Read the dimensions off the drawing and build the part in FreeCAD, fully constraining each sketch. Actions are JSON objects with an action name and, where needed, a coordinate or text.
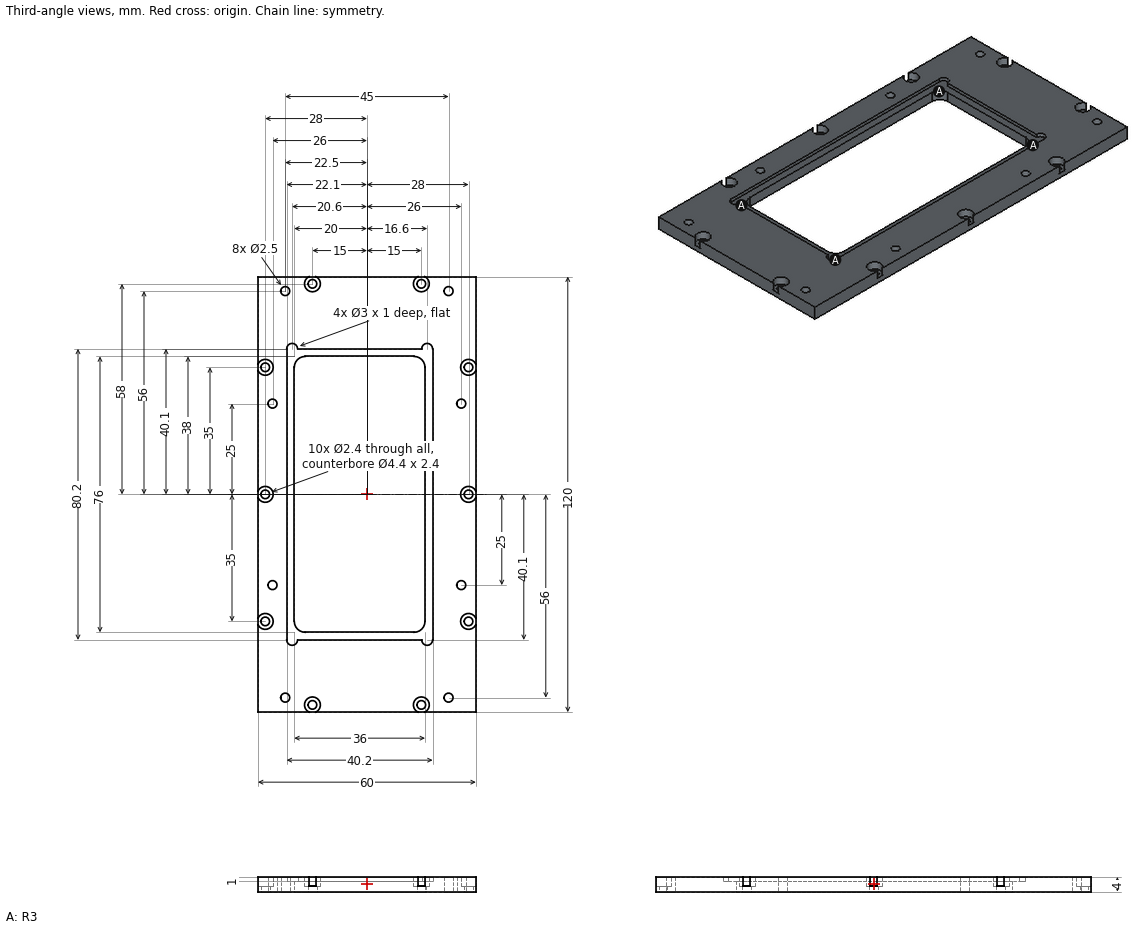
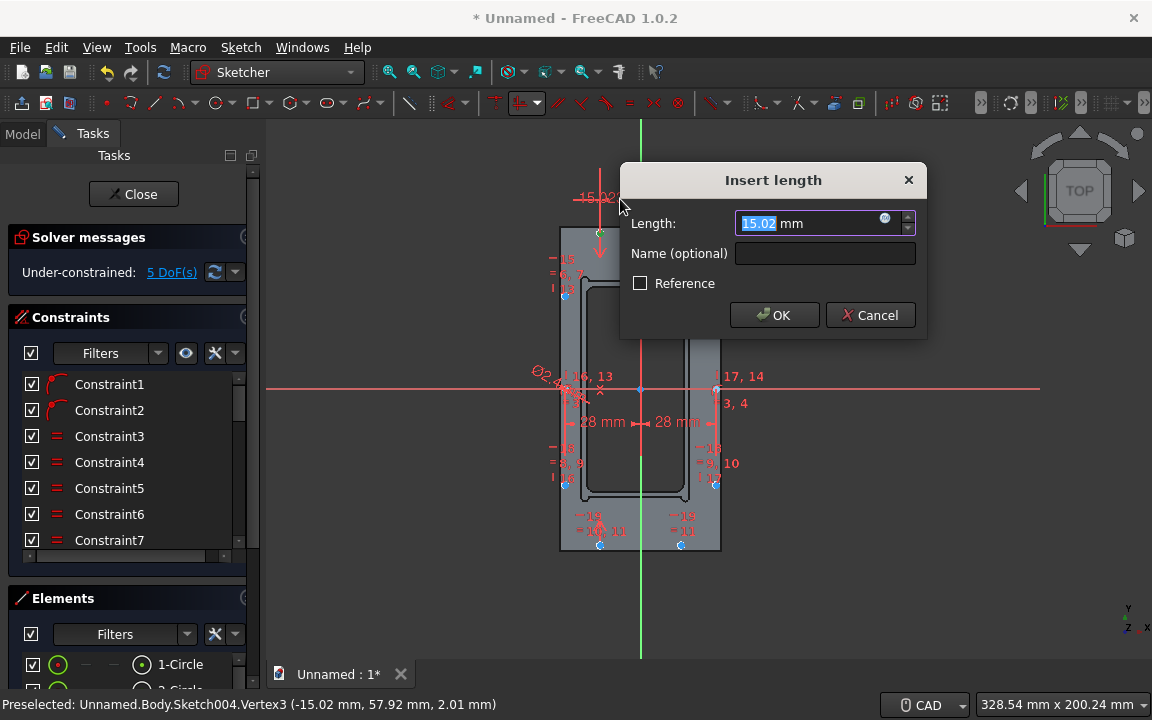
{"action": "type", "text": "15"}
{"action": "key", "text": "Return"}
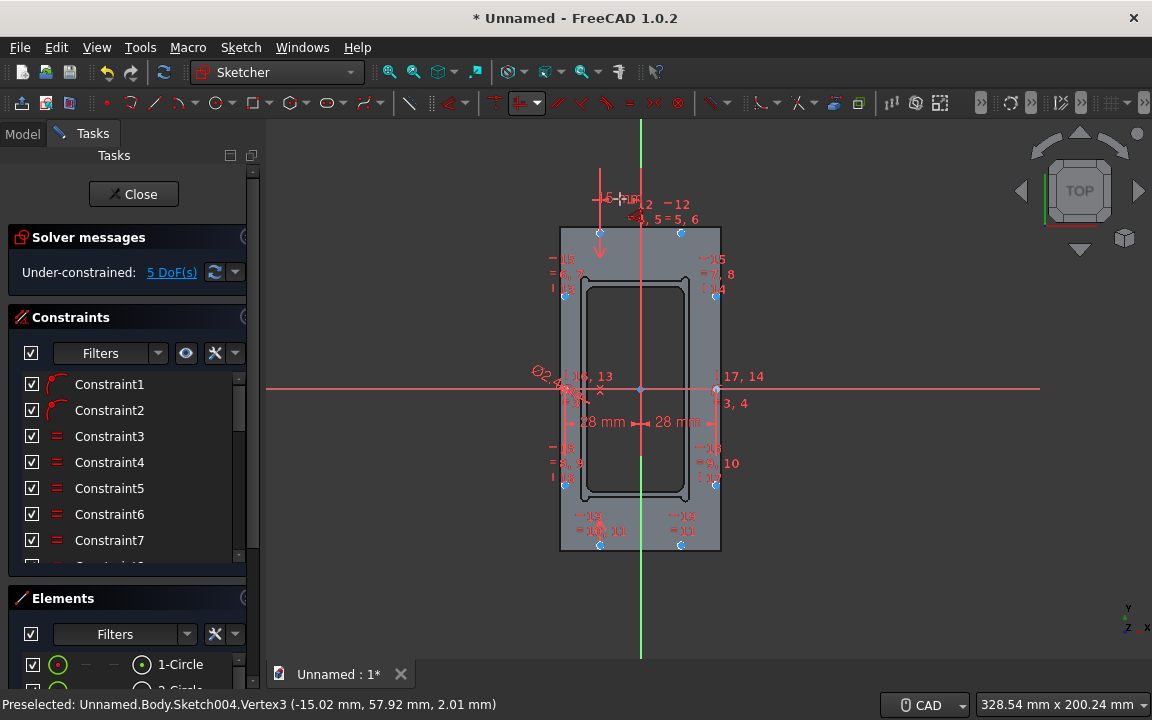
{"action": "left_click", "coordinate": [600, 233]}
{"action": "left_click", "coordinate": [566, 275]}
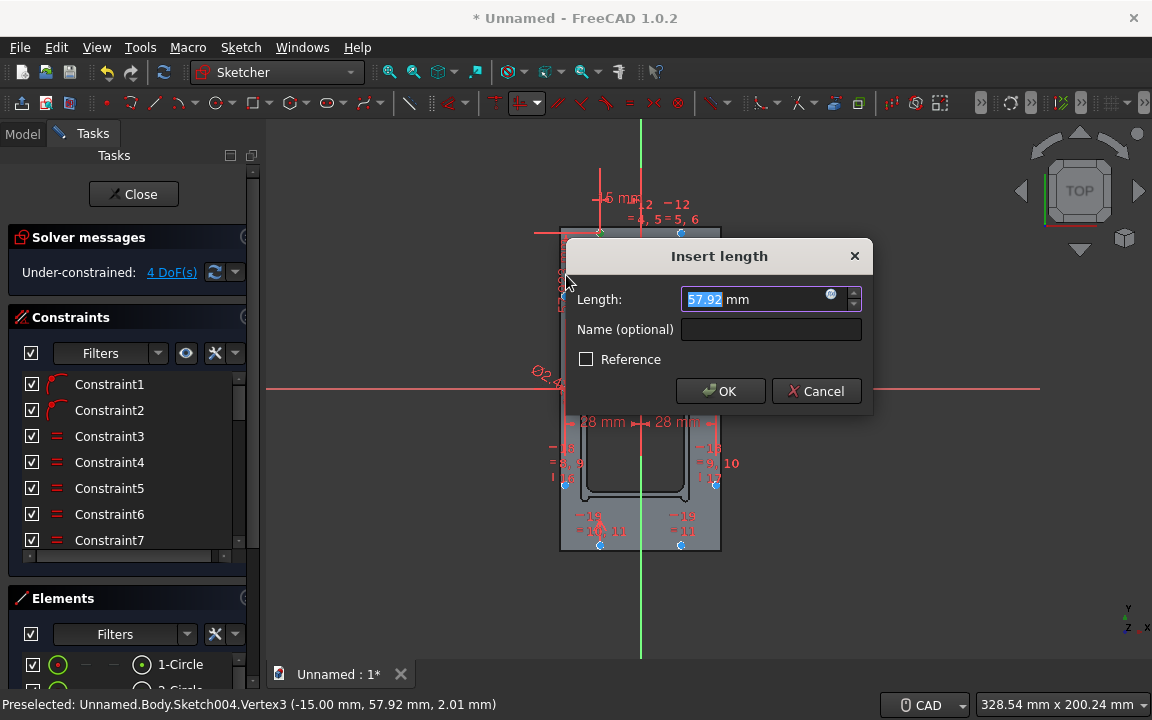
{"action": "type", "text": "58"}
{"action": "key", "text": "Return"}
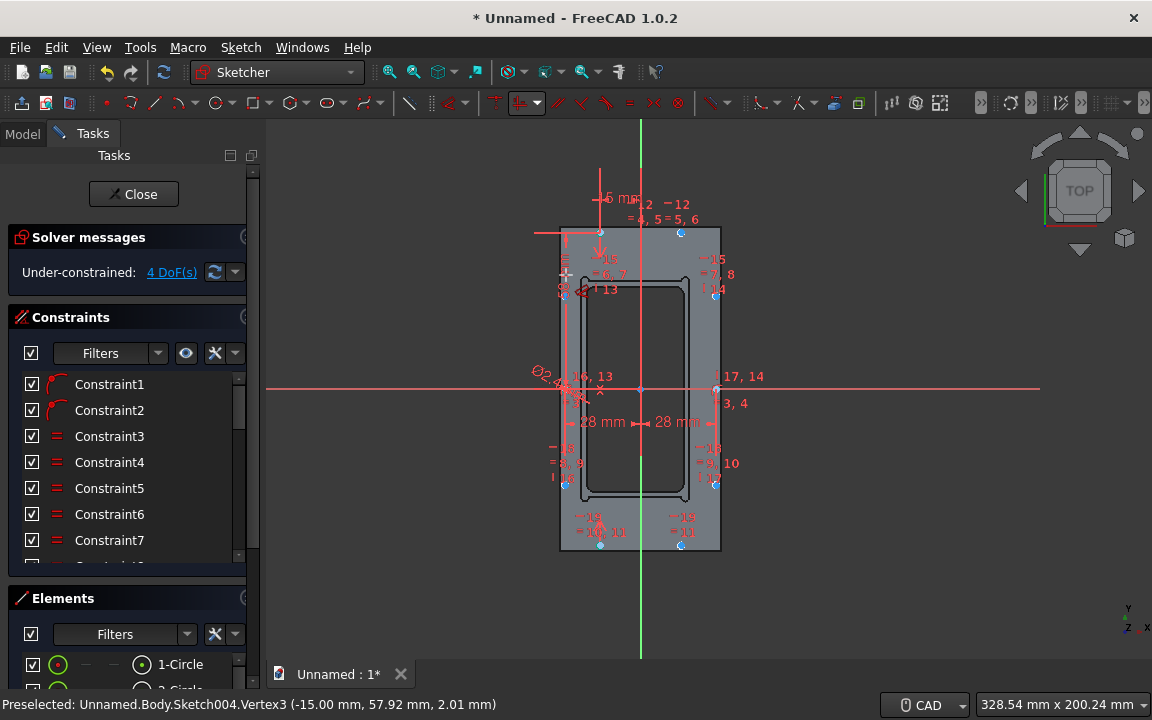
{"action": "left_click", "coordinate": [681, 233]}
{"action": "left_click", "coordinate": [661, 175]}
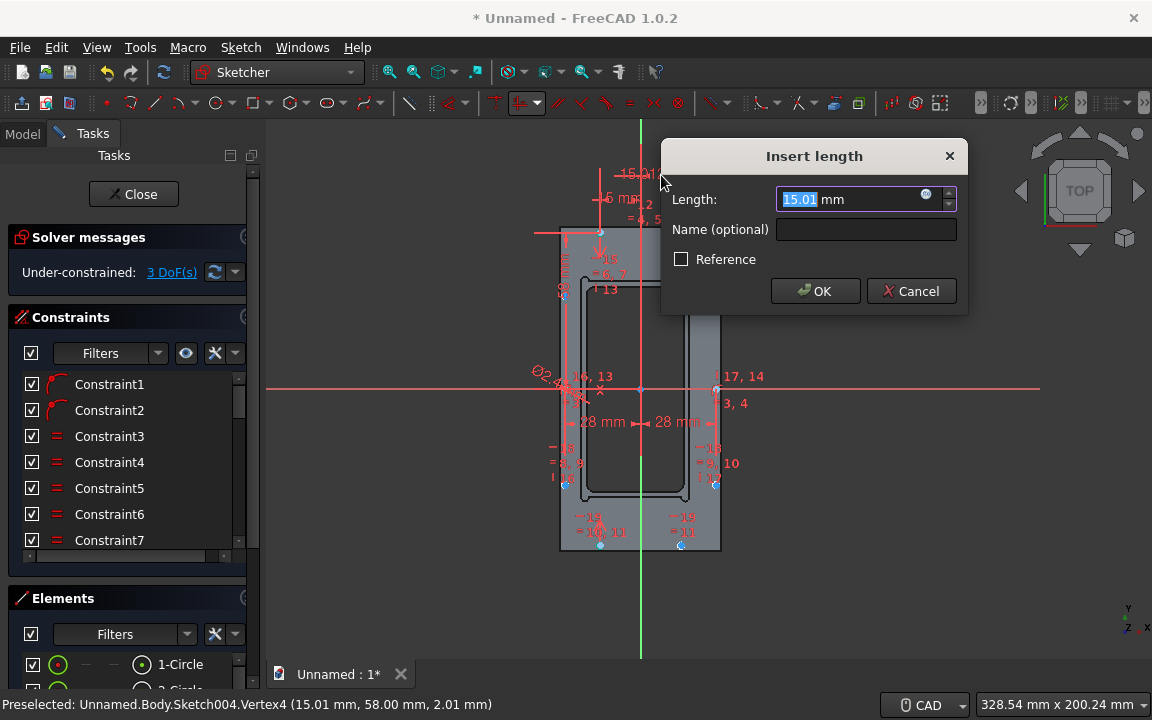
{"action": "type", "text": "15"}
{"action": "key", "text": "Return"}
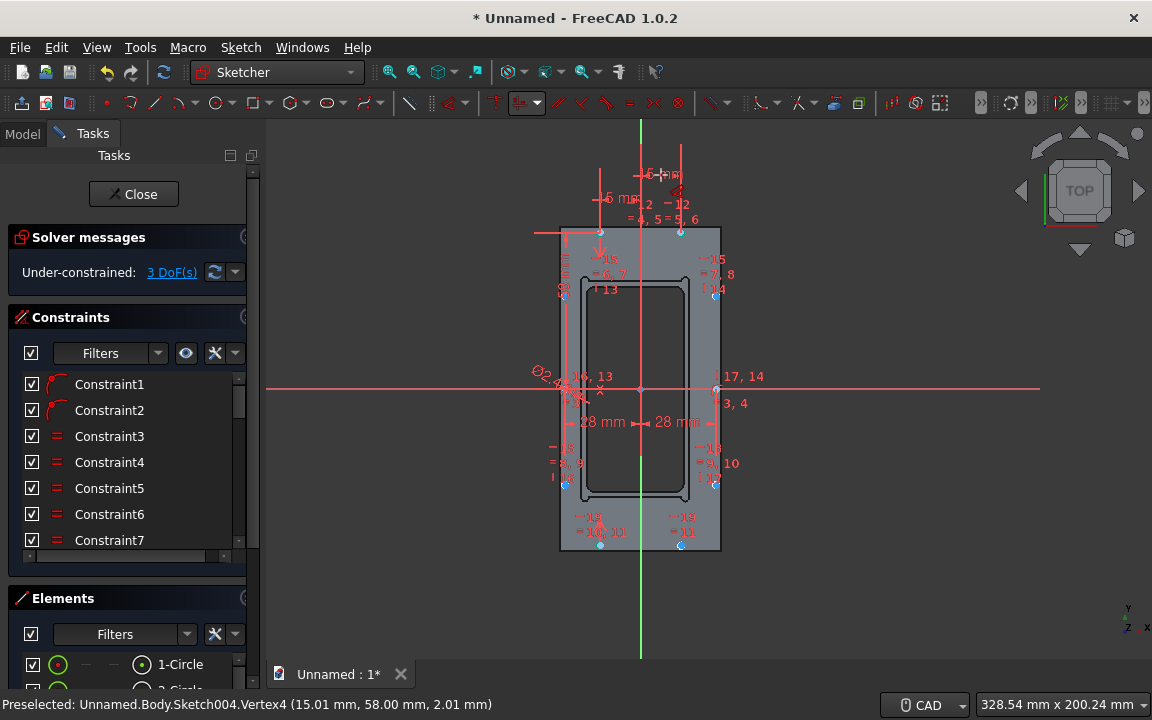
{"action": "left_click", "coordinate": [565, 296]}
{"action": "left_click", "coordinate": [531, 343]}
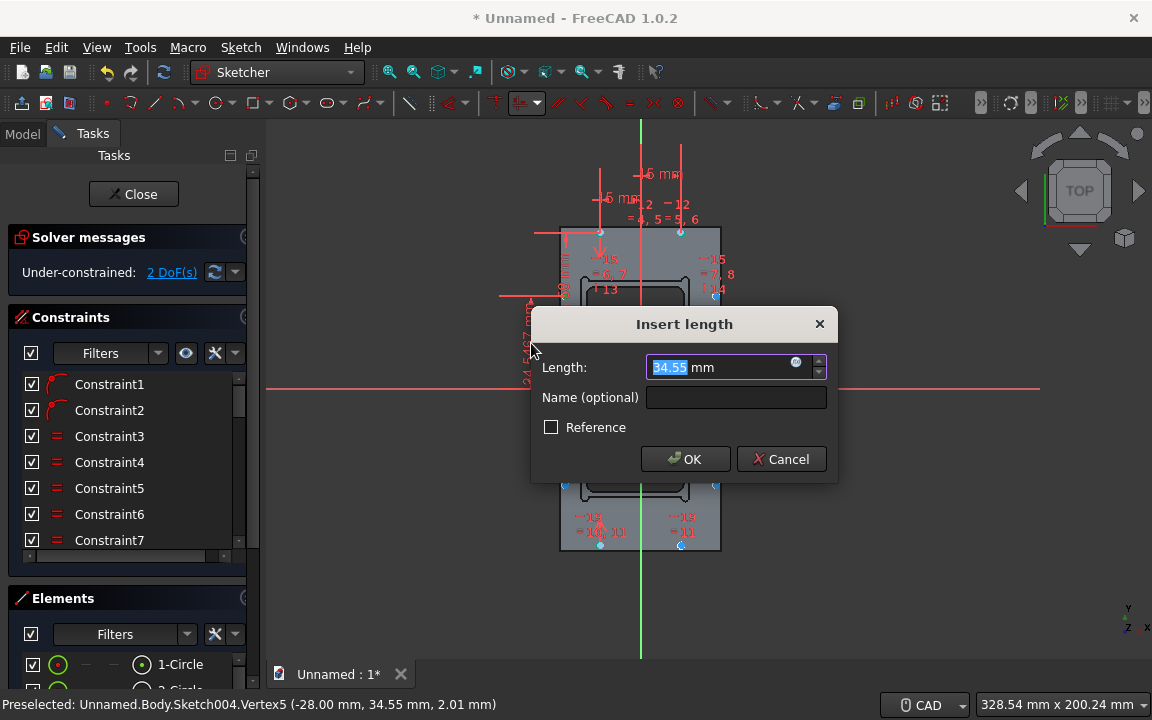
{"action": "type", "text": "35"}
{"action": "key", "text": "Return"}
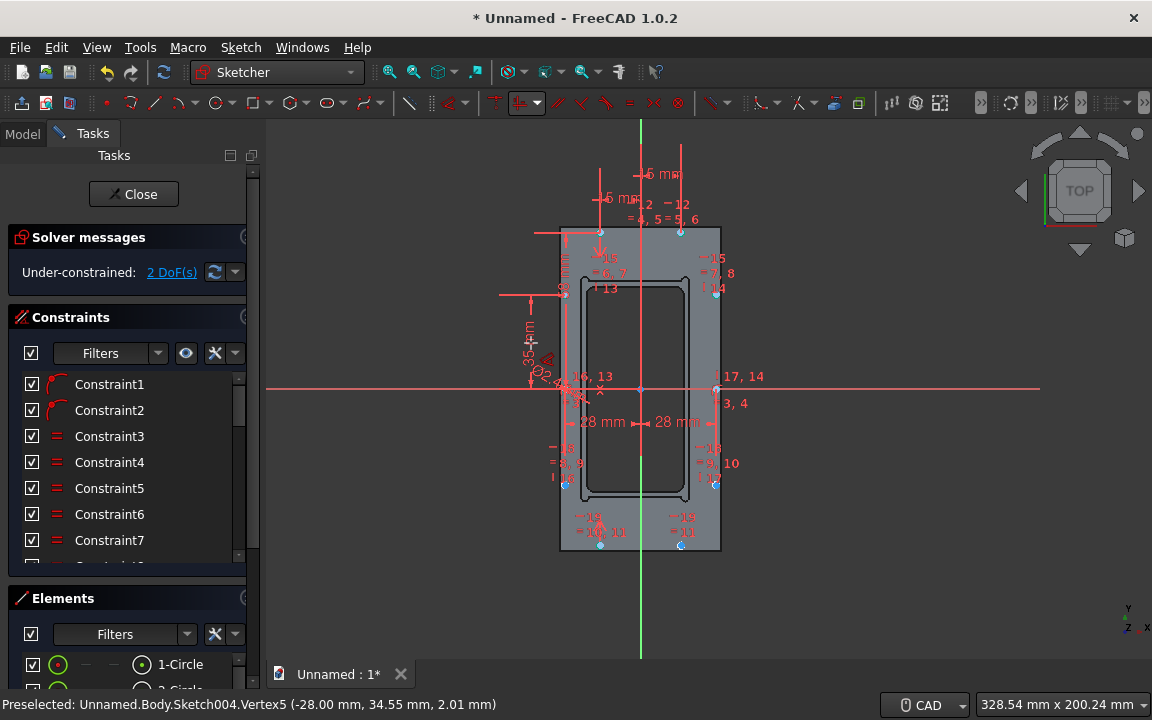
{"action": "left_click", "coordinate": [565, 485]}
{"action": "left_click", "coordinate": [531, 437]}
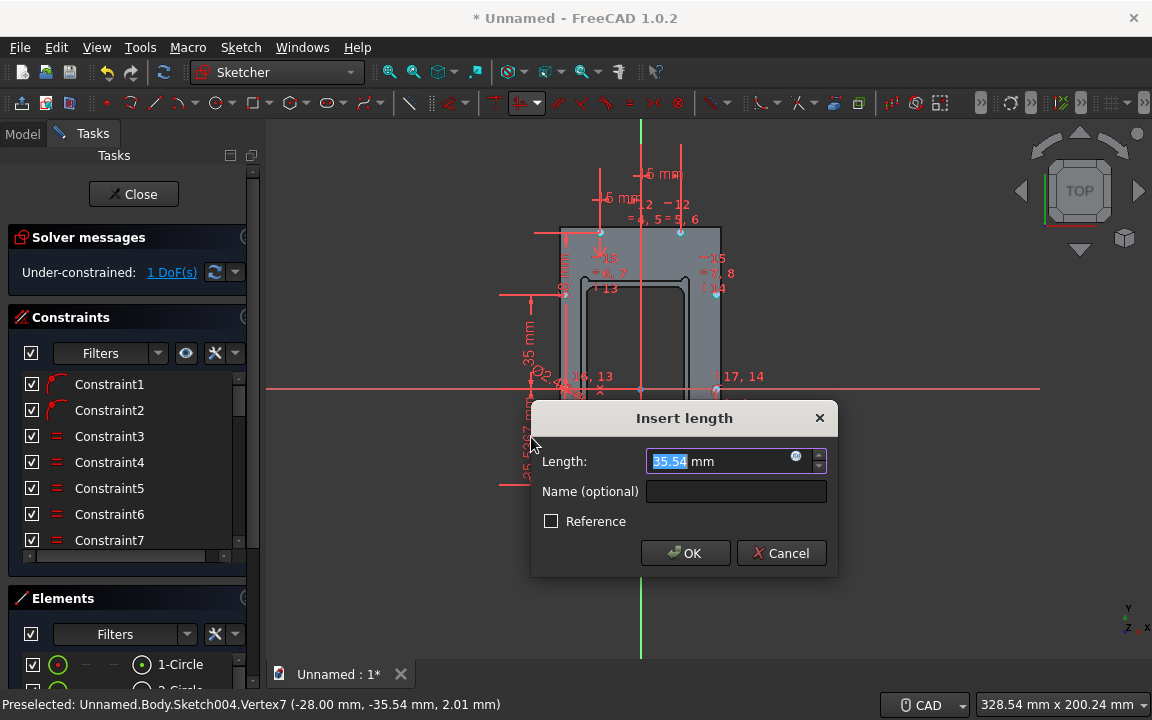
{"action": "type", "text": "35"}
{"action": "key", "text": "Return"}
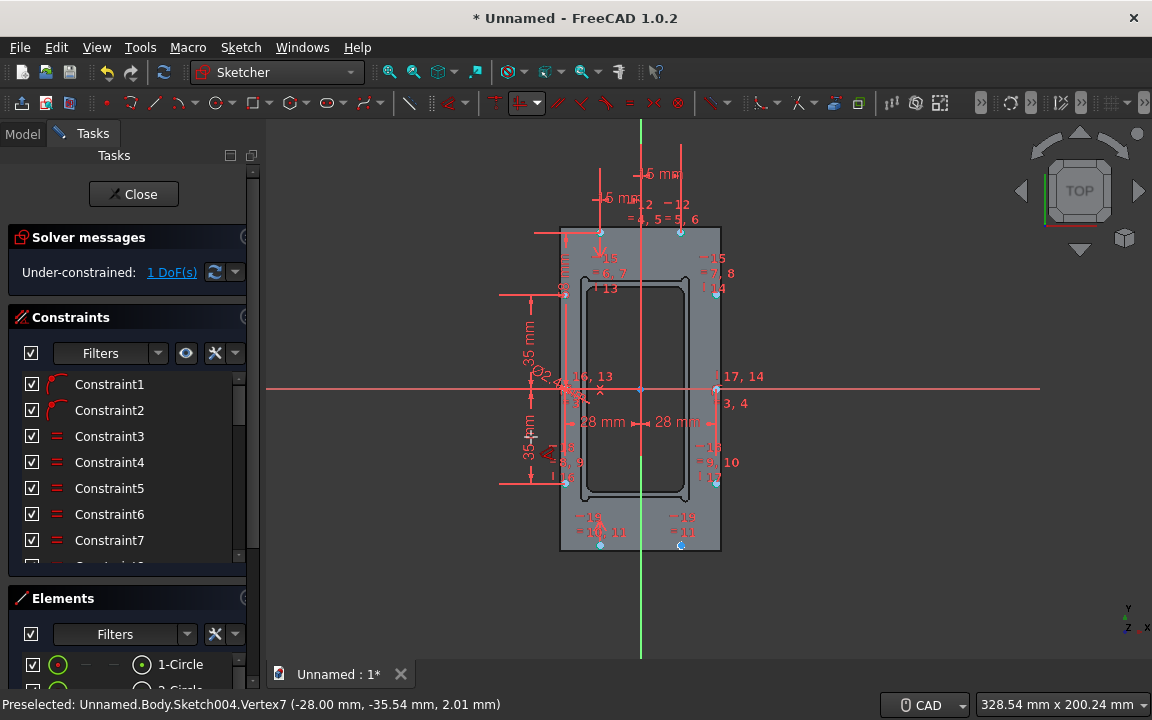
{"action": "left_click", "coordinate": [681, 546]}
{"action": "left_click", "coordinate": [661, 580]}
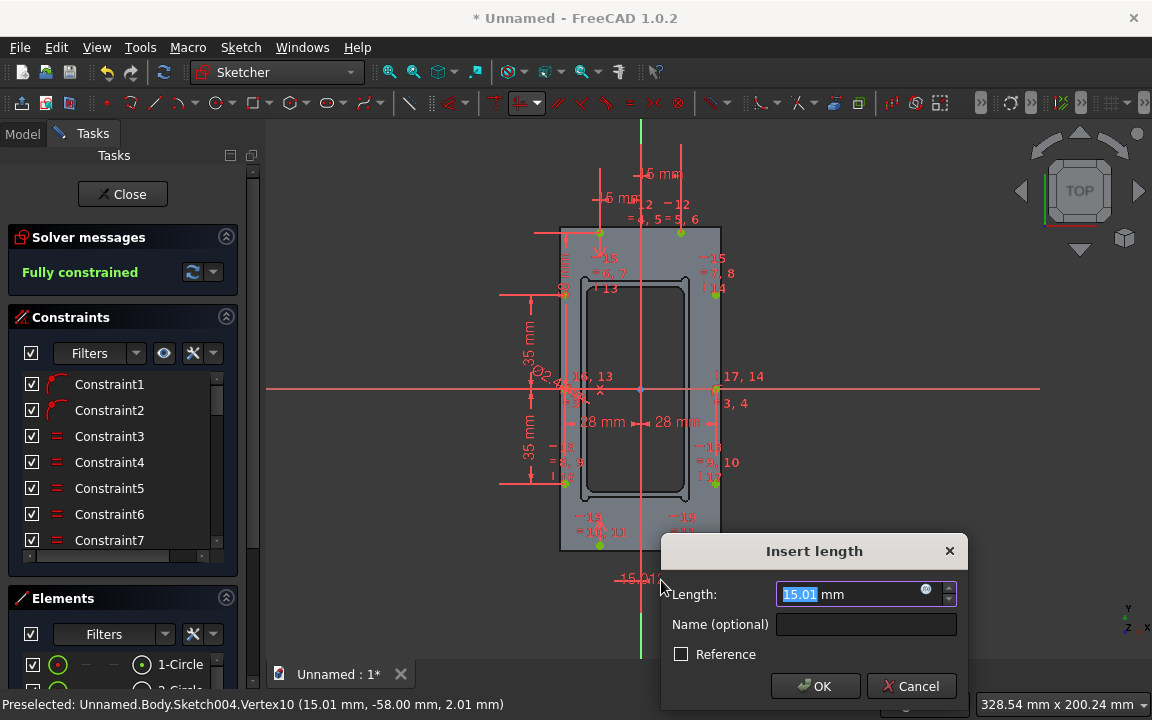
{"action": "type", "text": "15"}
{"action": "key", "text": "Return"}
{"action": "key", "text": "Escape"}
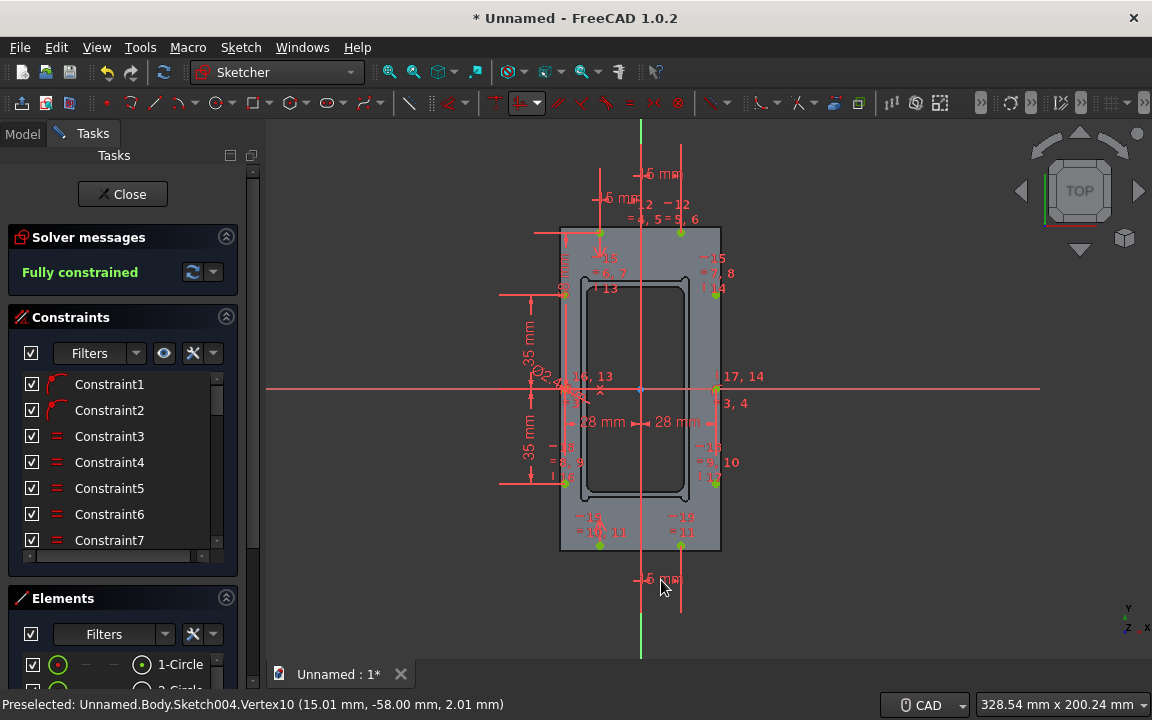
{"action": "left_click", "coordinate": [123, 194]}